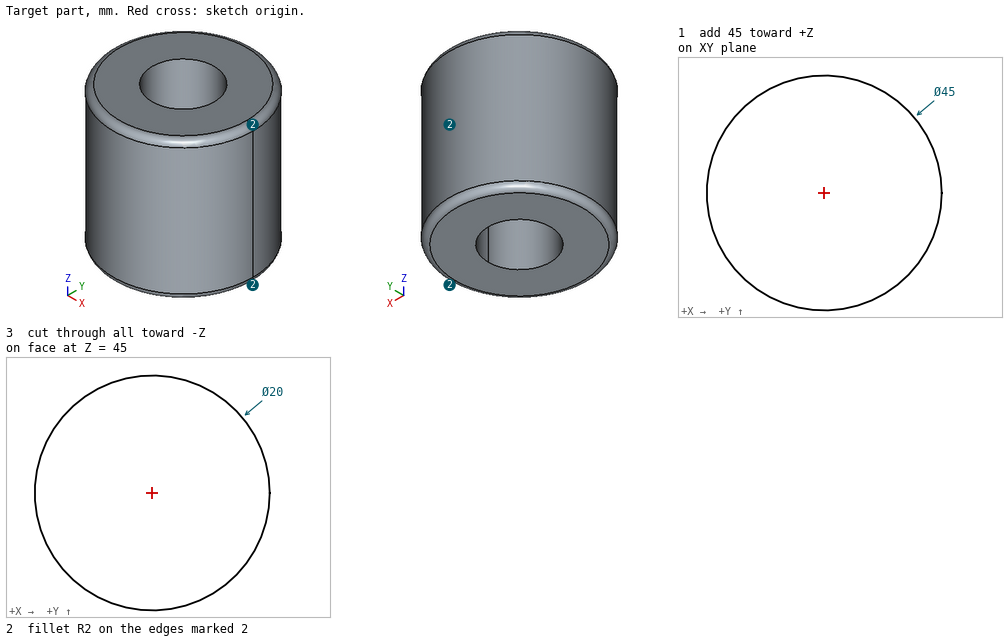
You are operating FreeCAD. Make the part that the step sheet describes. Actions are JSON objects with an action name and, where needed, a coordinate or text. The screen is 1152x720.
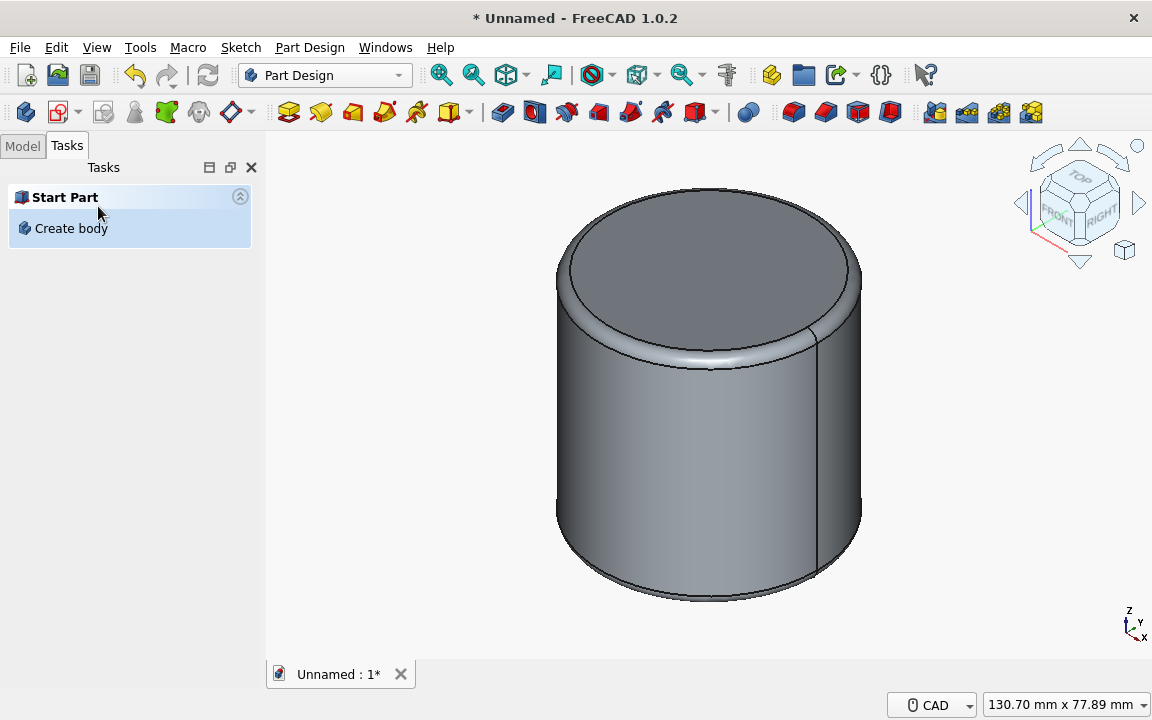
{"action": "left_click", "coordinate": [709, 269]}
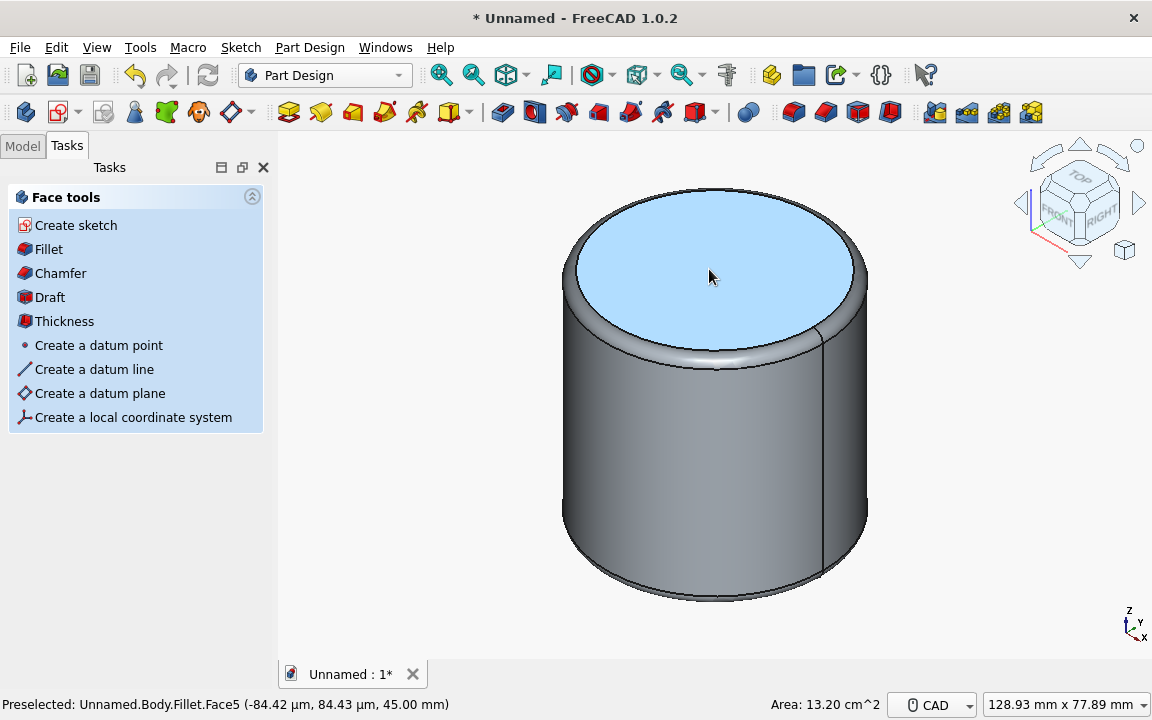
{"action": "left_click", "coordinate": [58, 112]}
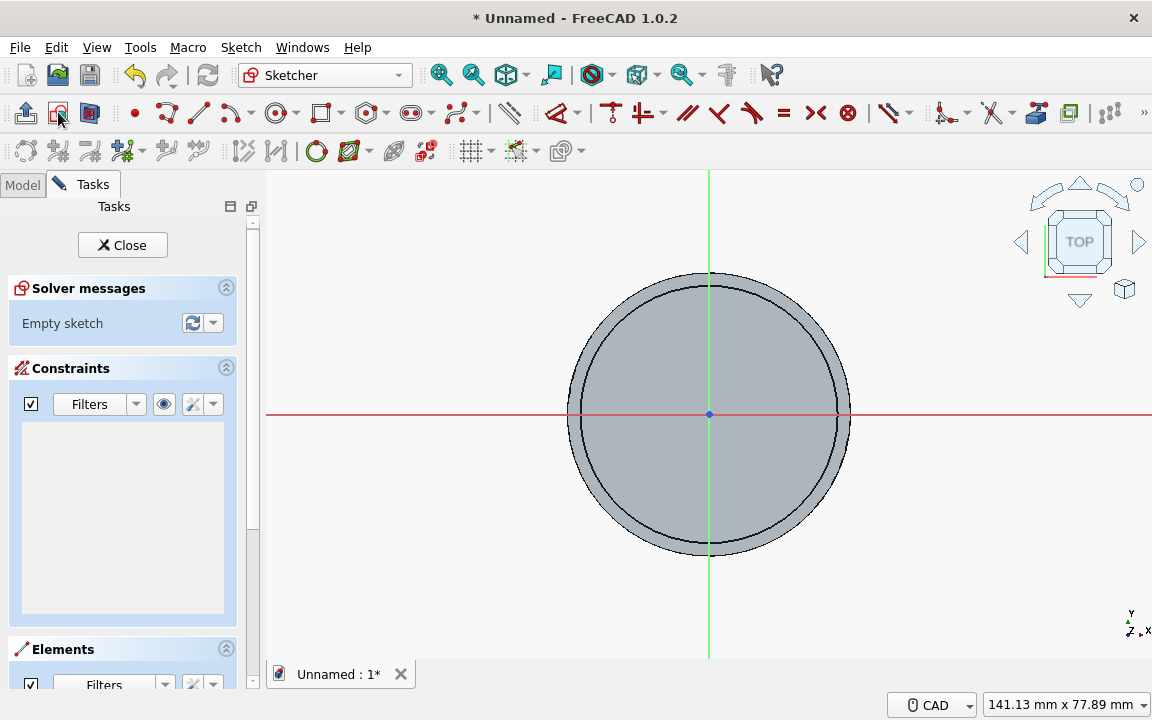
{"action": "scroll", "coordinate": [765, 414], "scroll_direction": "up", "scroll_amount": 4}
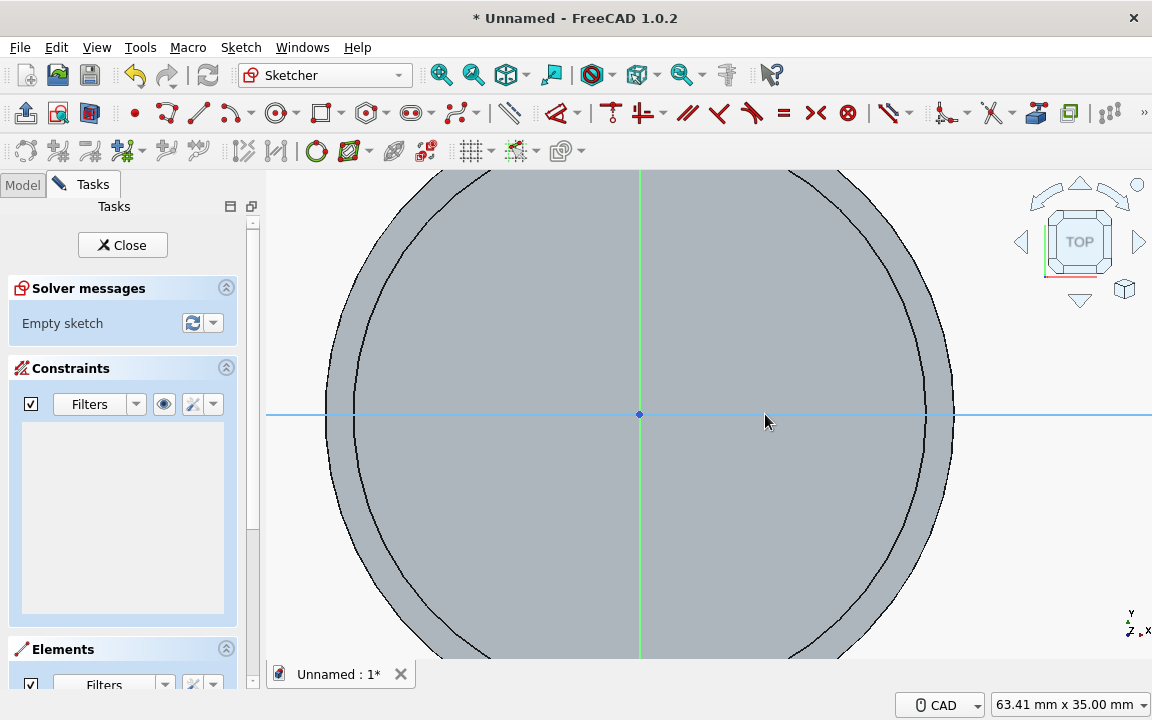
{"action": "left_click", "coordinate": [276, 114]}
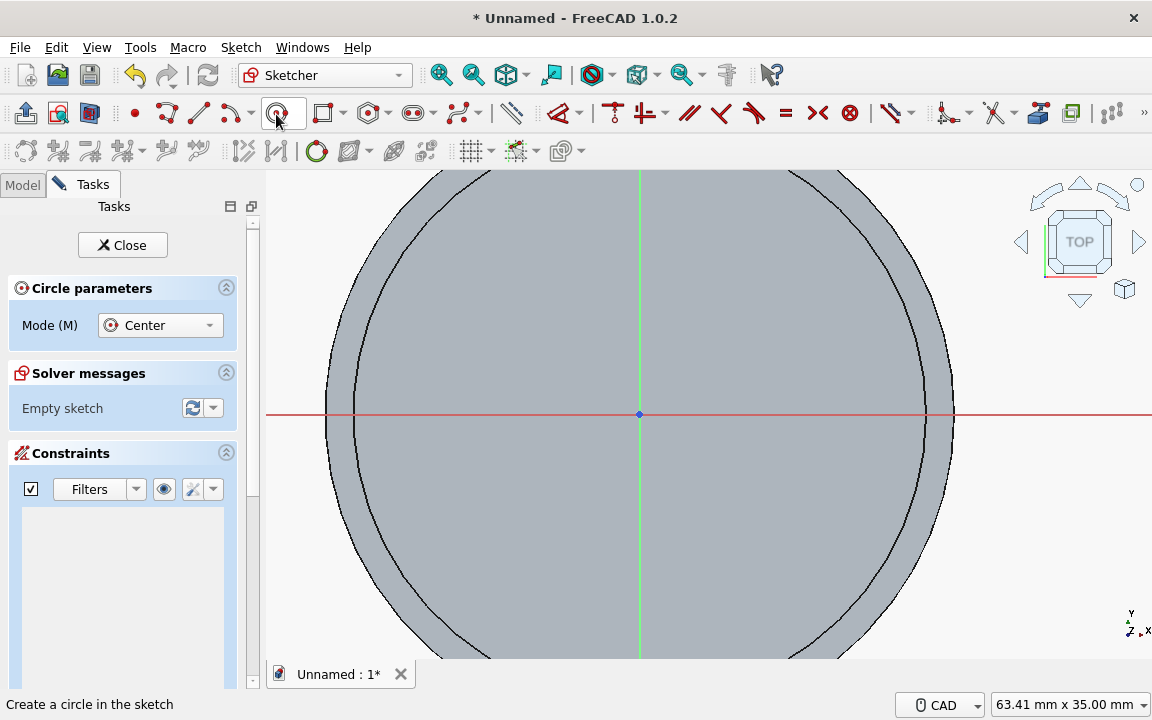
{"action": "left_click", "coordinate": [640, 414]}
{"action": "left_click", "coordinate": [738, 316]}
{"action": "key", "text": "Escape"}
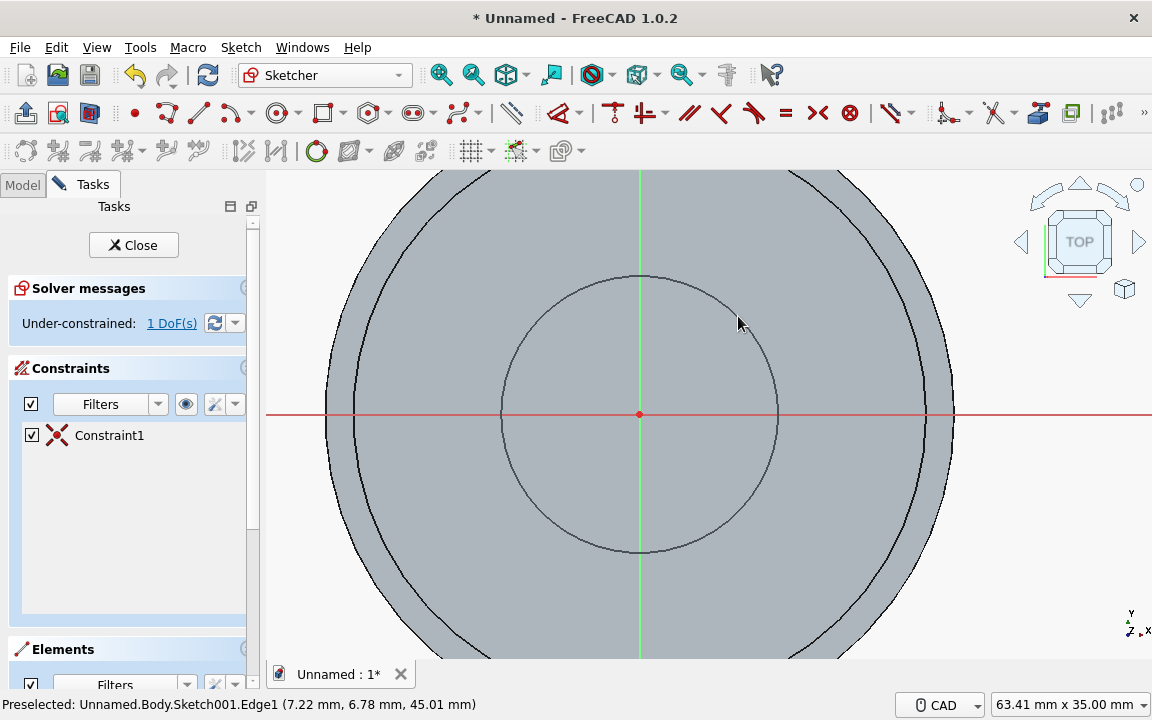
{"action": "left_click", "coordinate": [558, 114]}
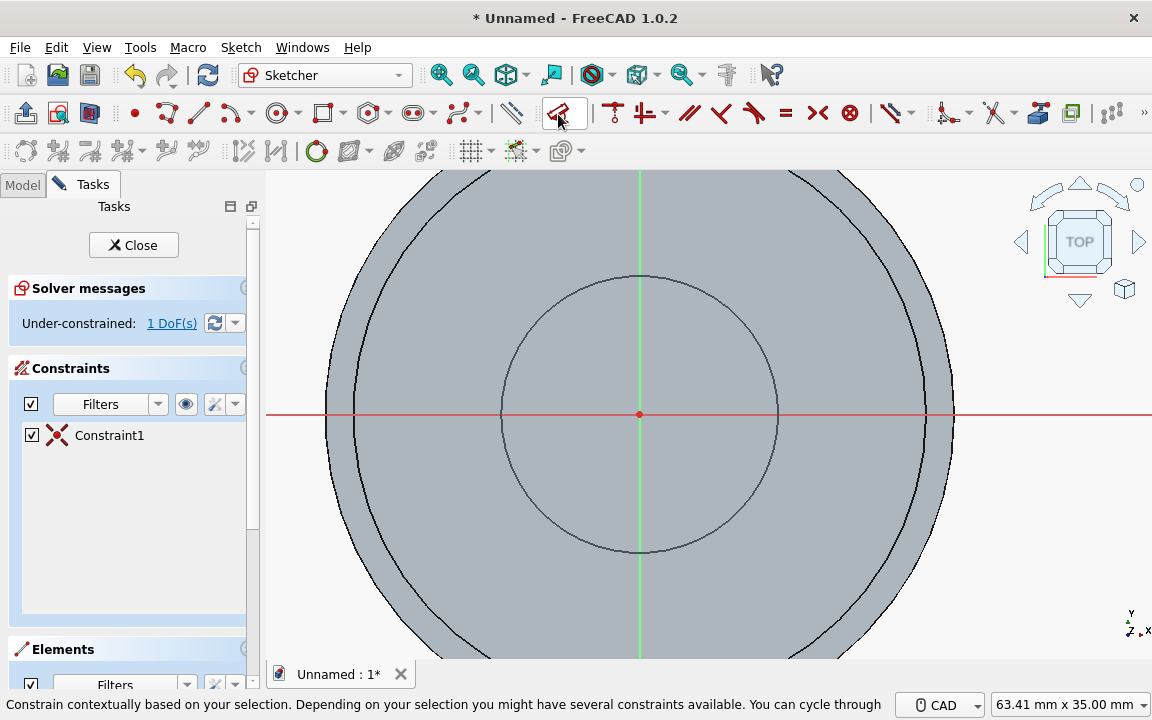
{"action": "left_click", "coordinate": [737, 316]}
{"action": "left_click", "coordinate": [759, 293]}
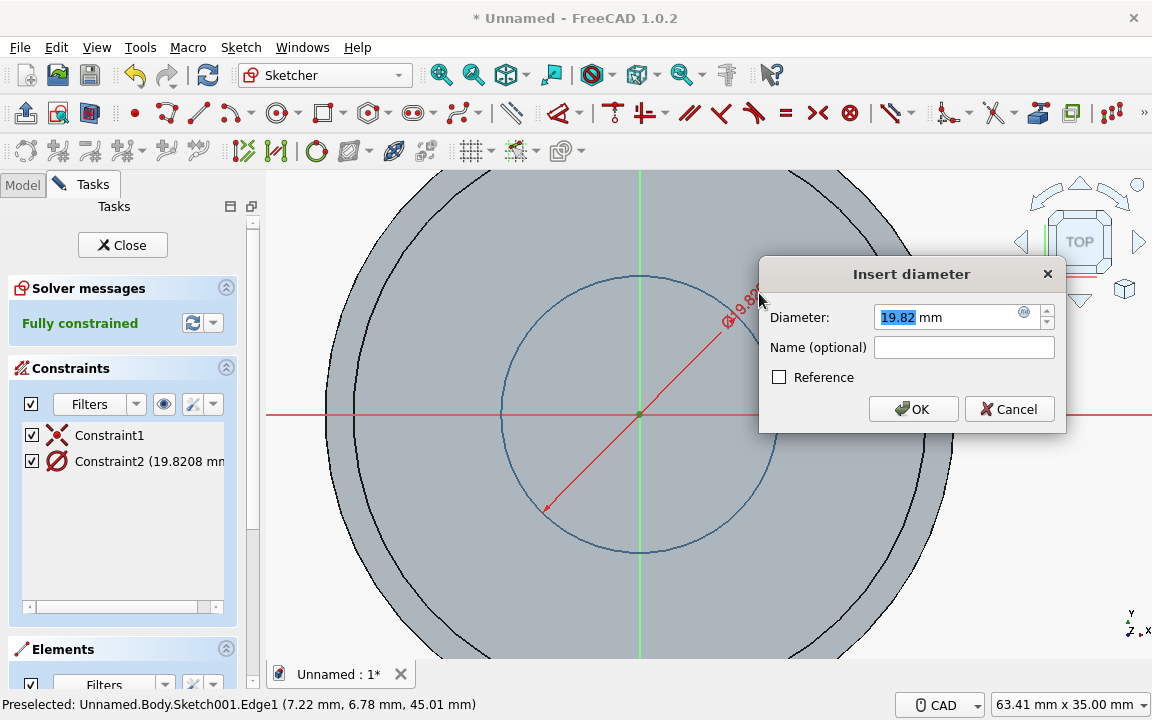
{"action": "type", "text": "20"}
{"action": "key", "text": "Return"}
{"action": "key", "text": "Escape"}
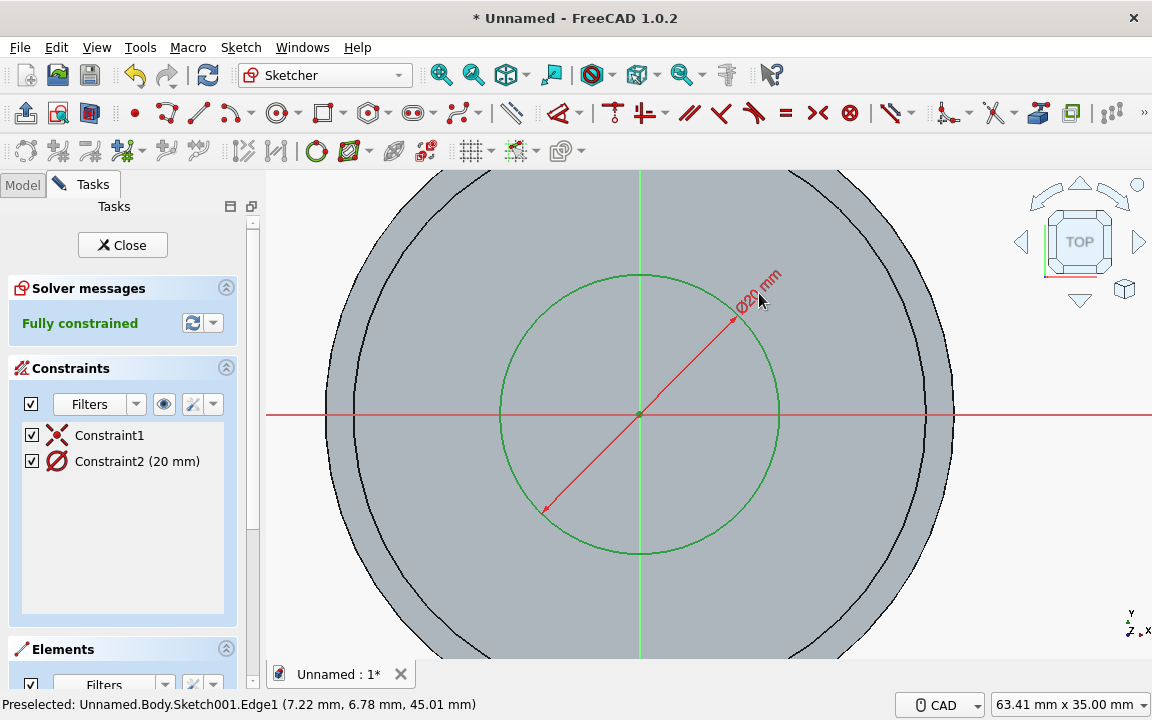
{"action": "left_click", "coordinate": [123, 245]}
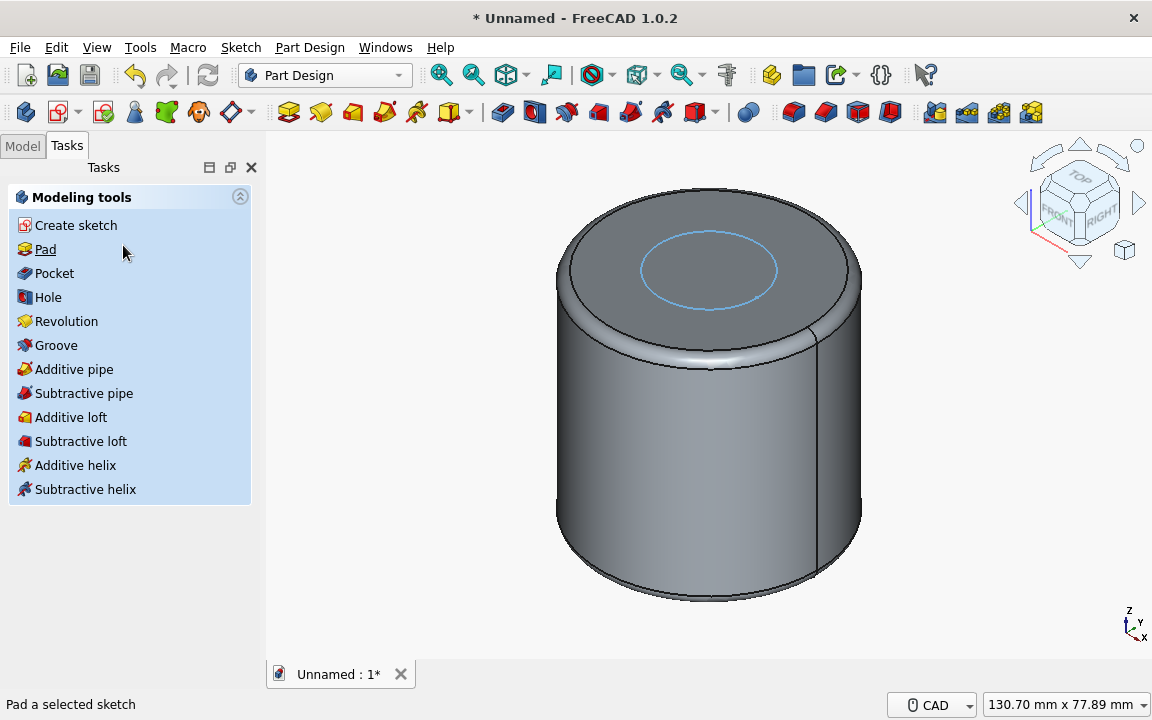
{"action": "left_click", "coordinate": [504, 112]}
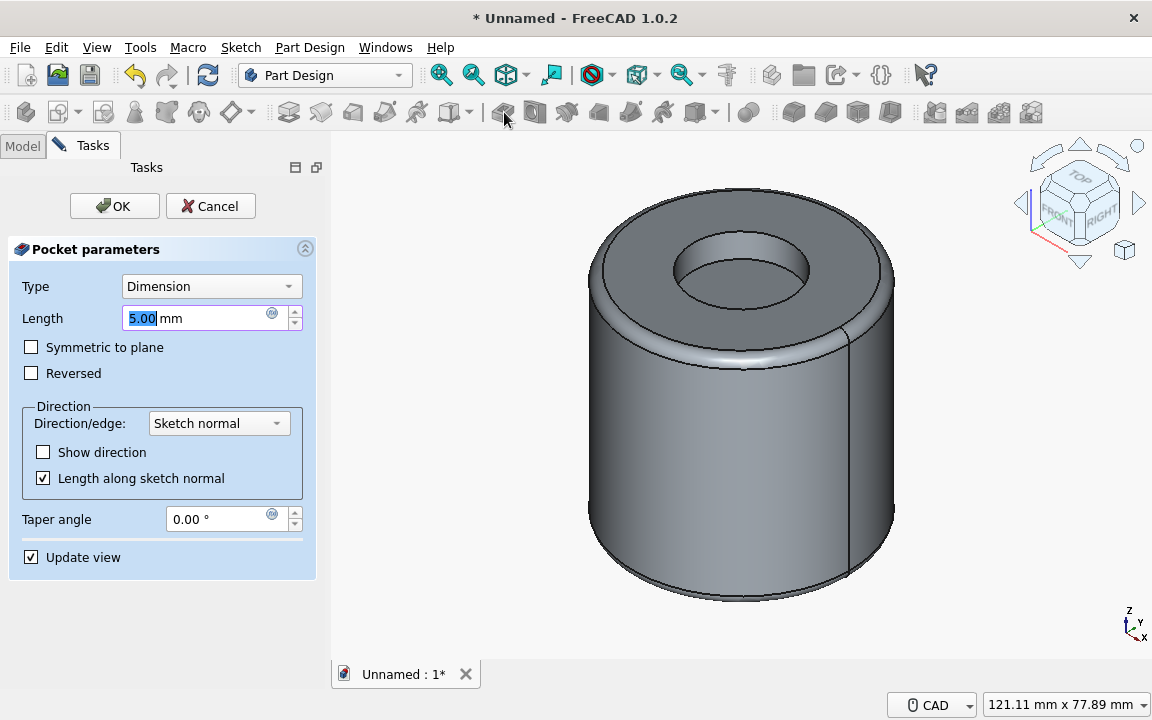
{"action": "left_click", "coordinate": [212, 286]}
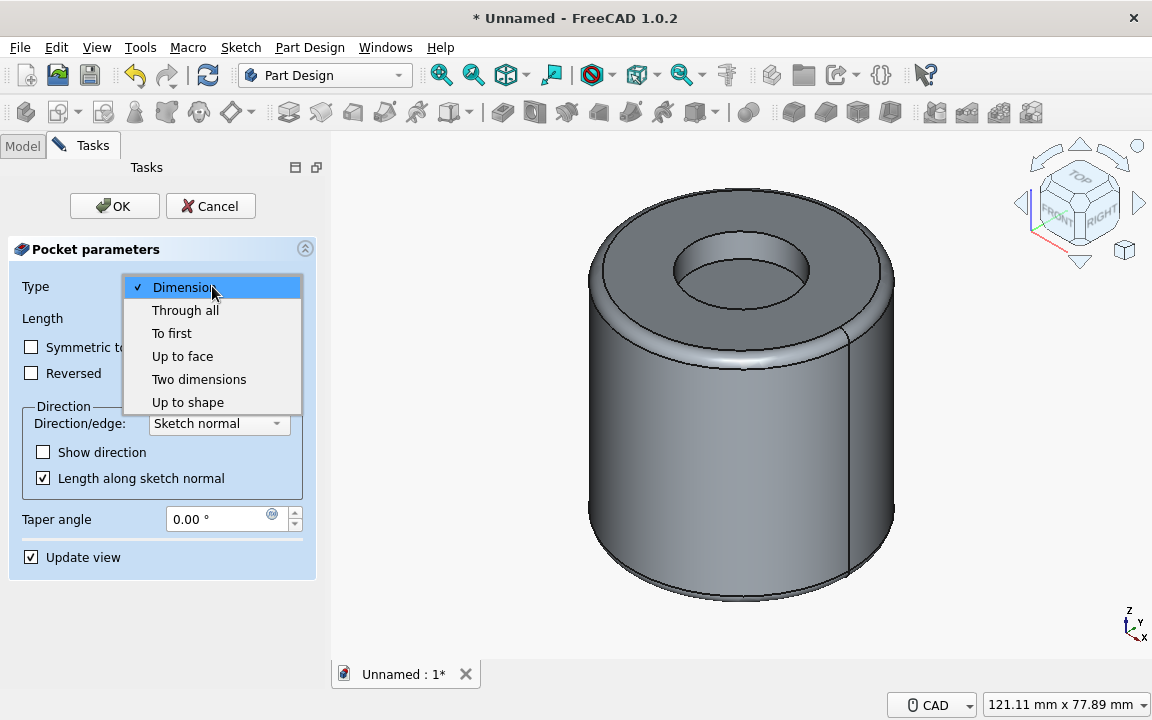
{"action": "left_click", "coordinate": [212, 310]}